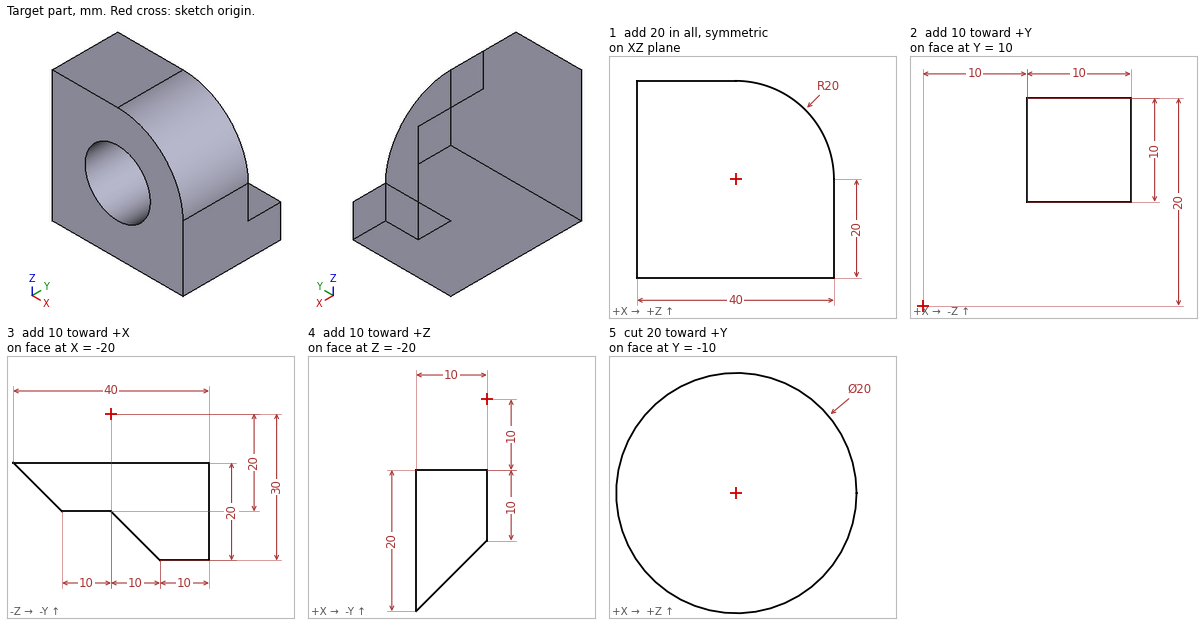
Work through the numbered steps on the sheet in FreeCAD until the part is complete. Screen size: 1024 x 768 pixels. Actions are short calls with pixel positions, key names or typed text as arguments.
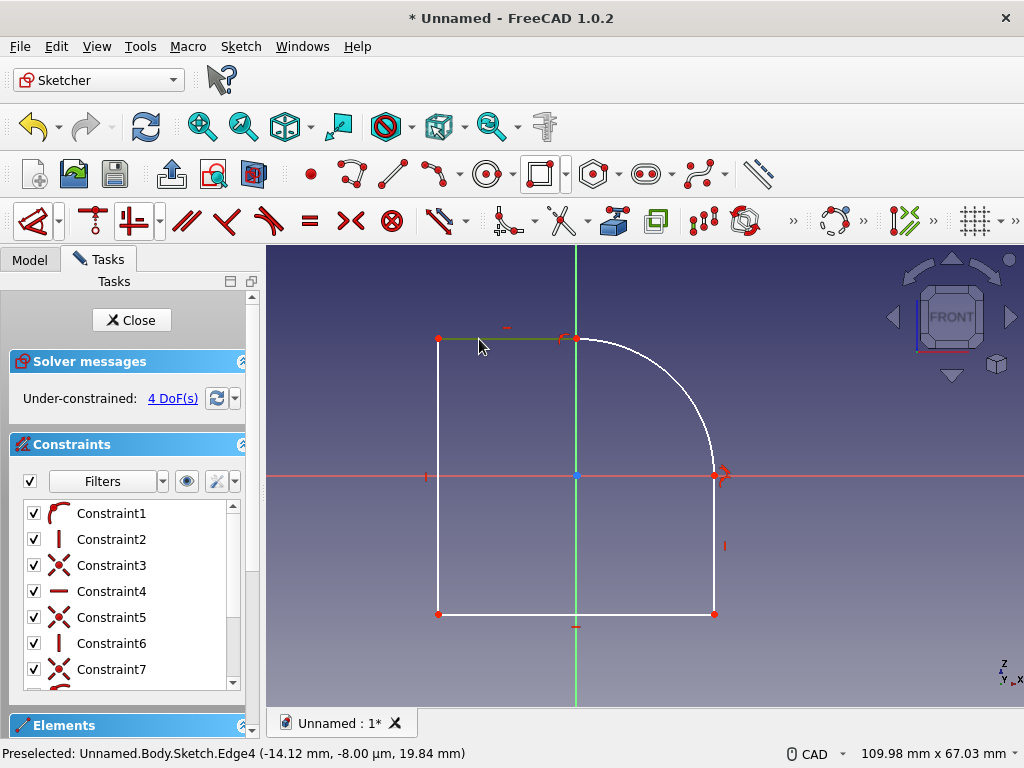
click(699, 413)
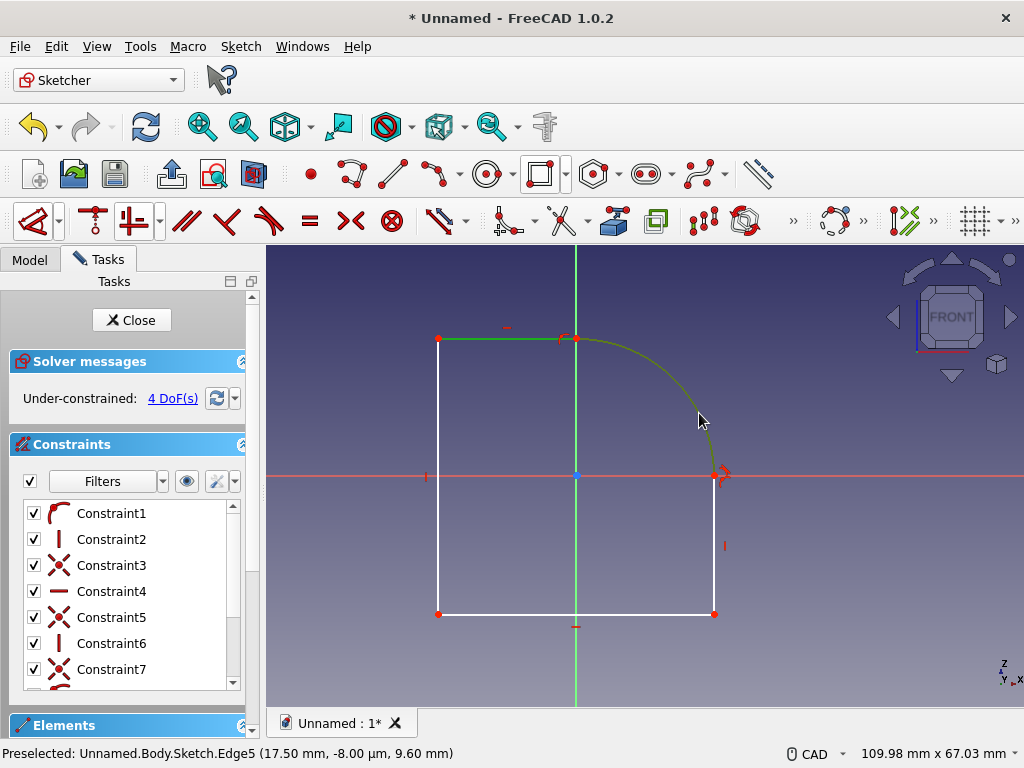
click(269, 222)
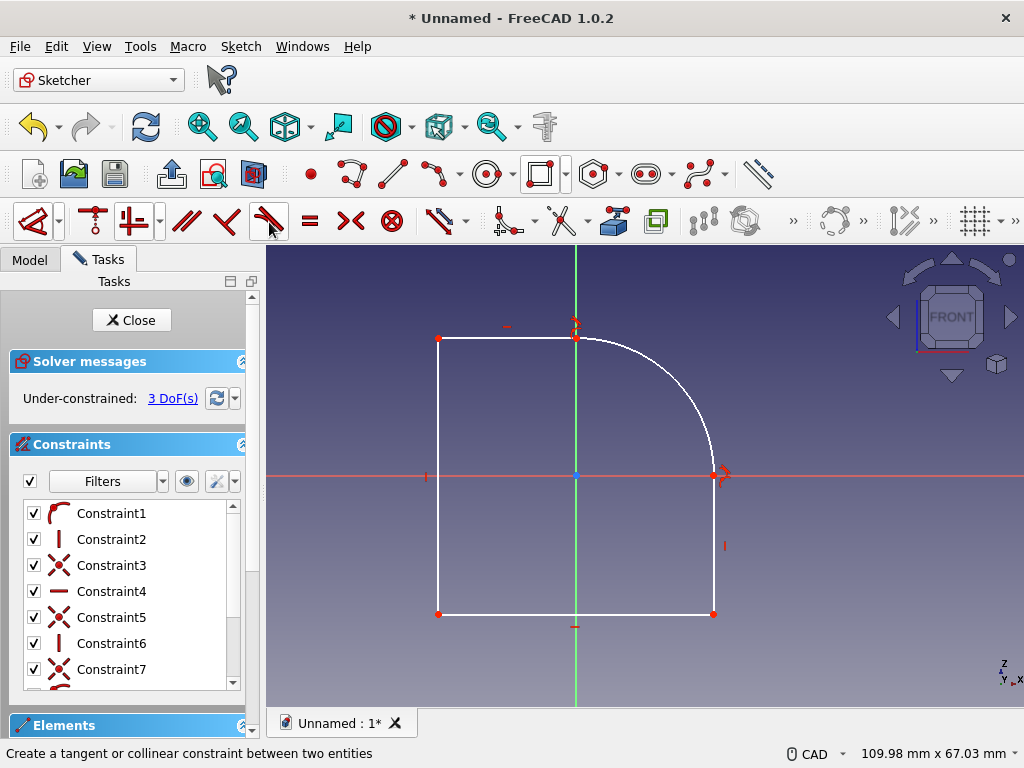
click(699, 413)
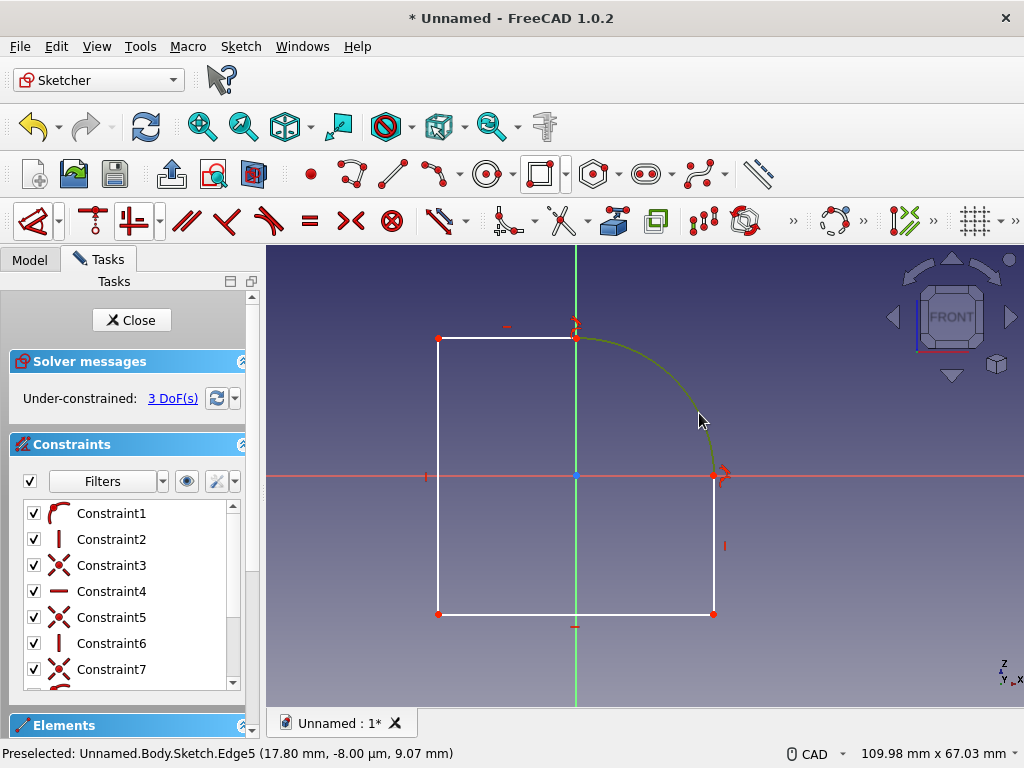
key(k)
key(r)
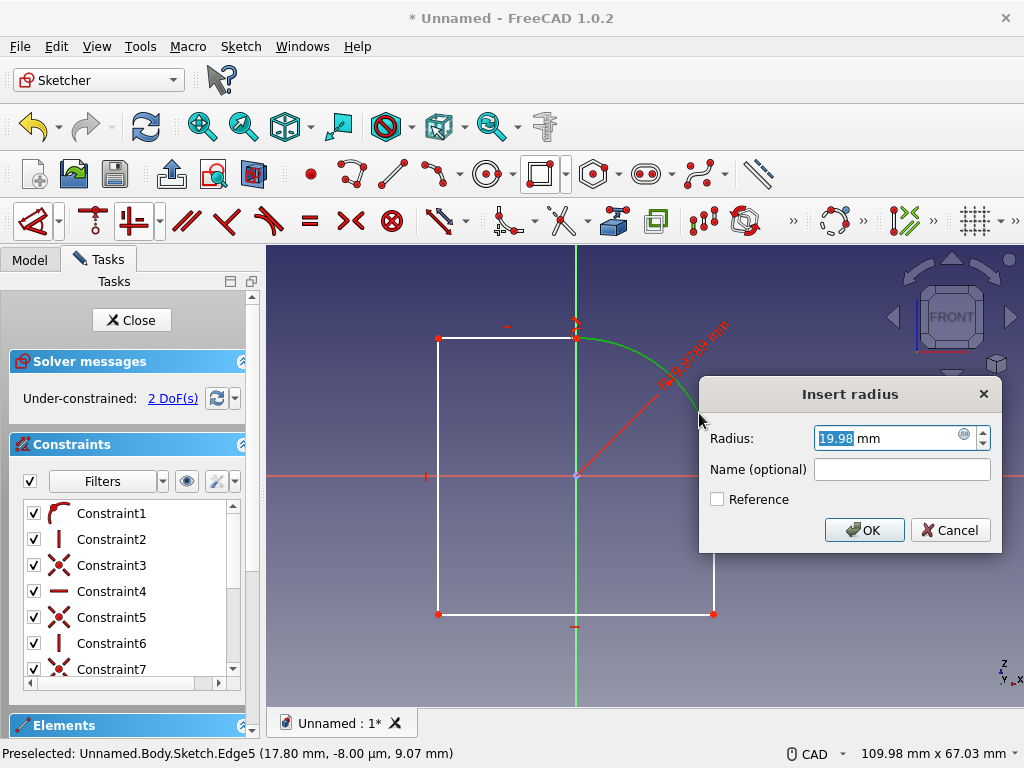
text(20)
key(Return)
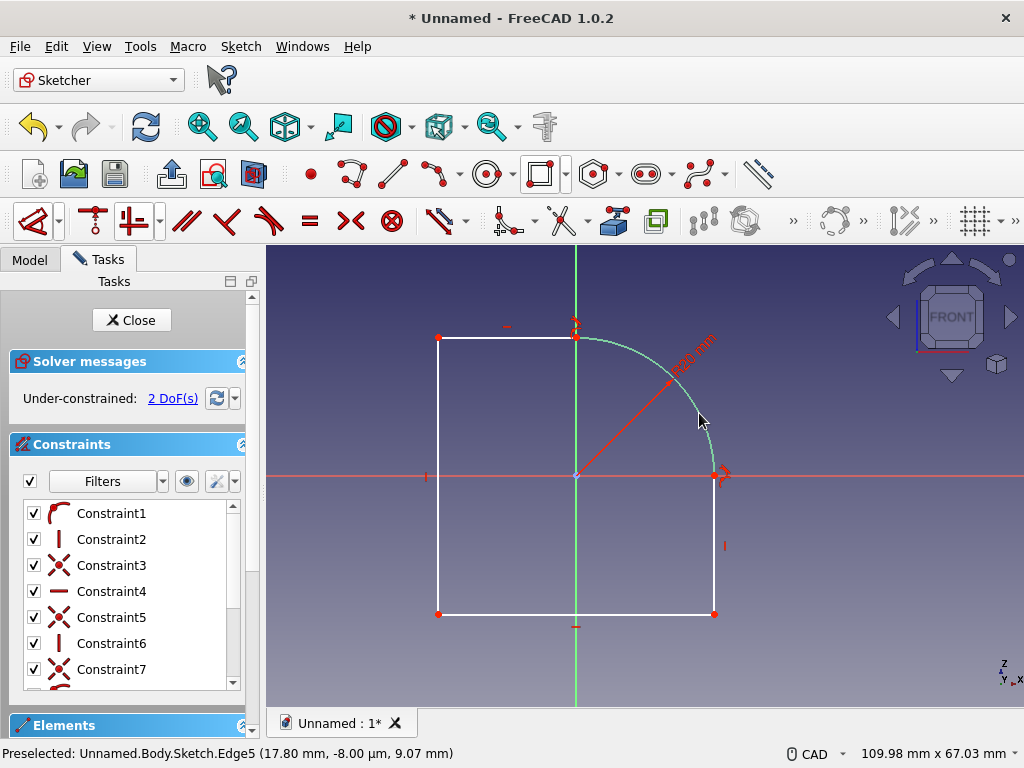
click(714, 518)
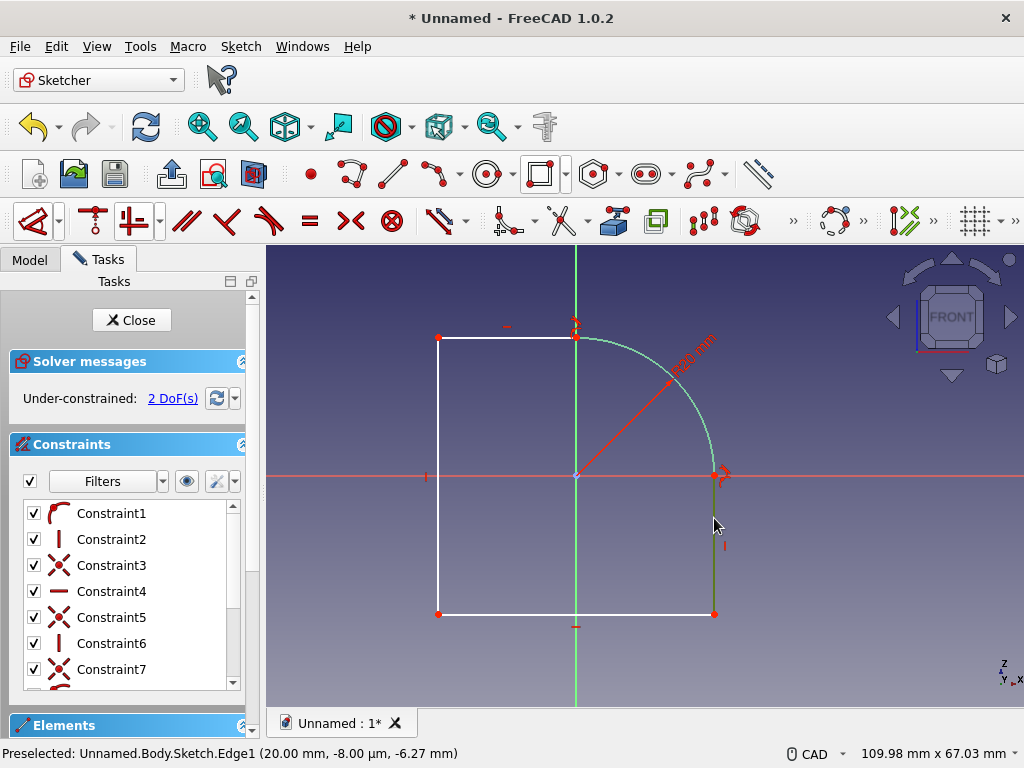
click(58, 222)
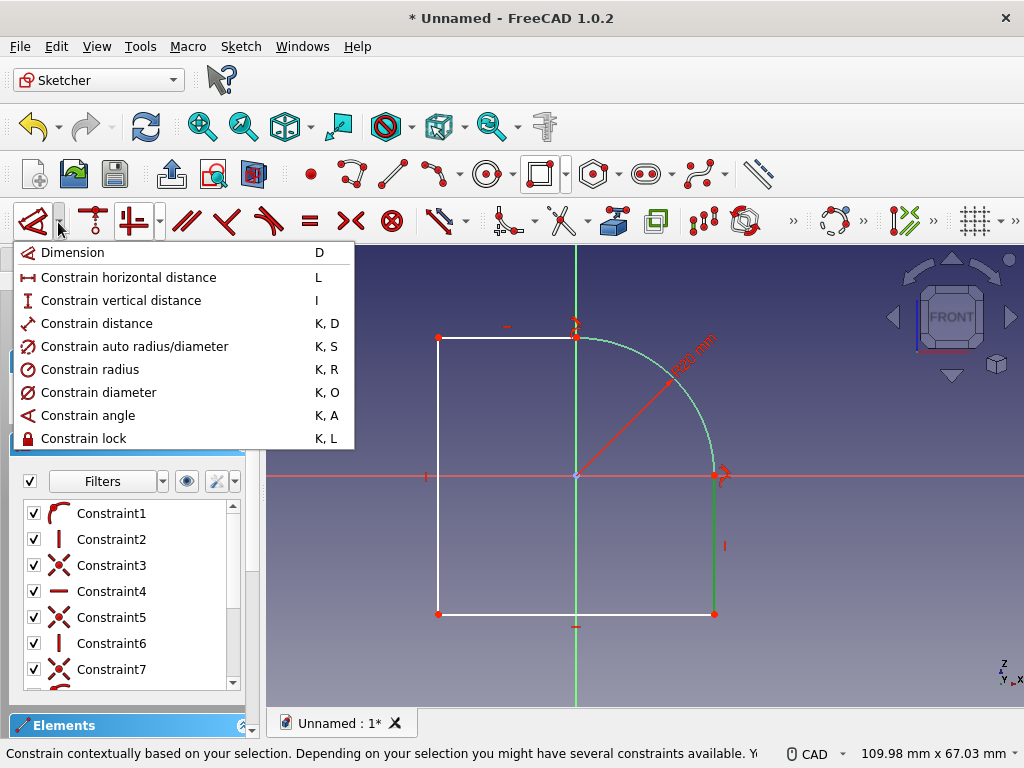
click(184, 300)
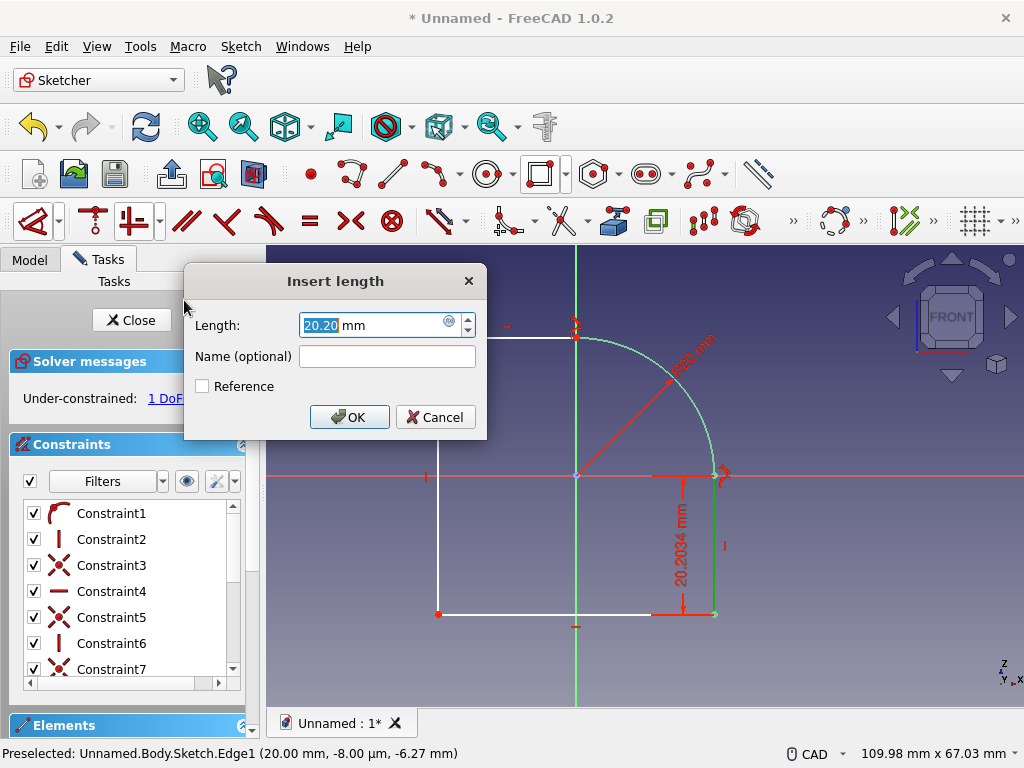
text(20)
key(Return)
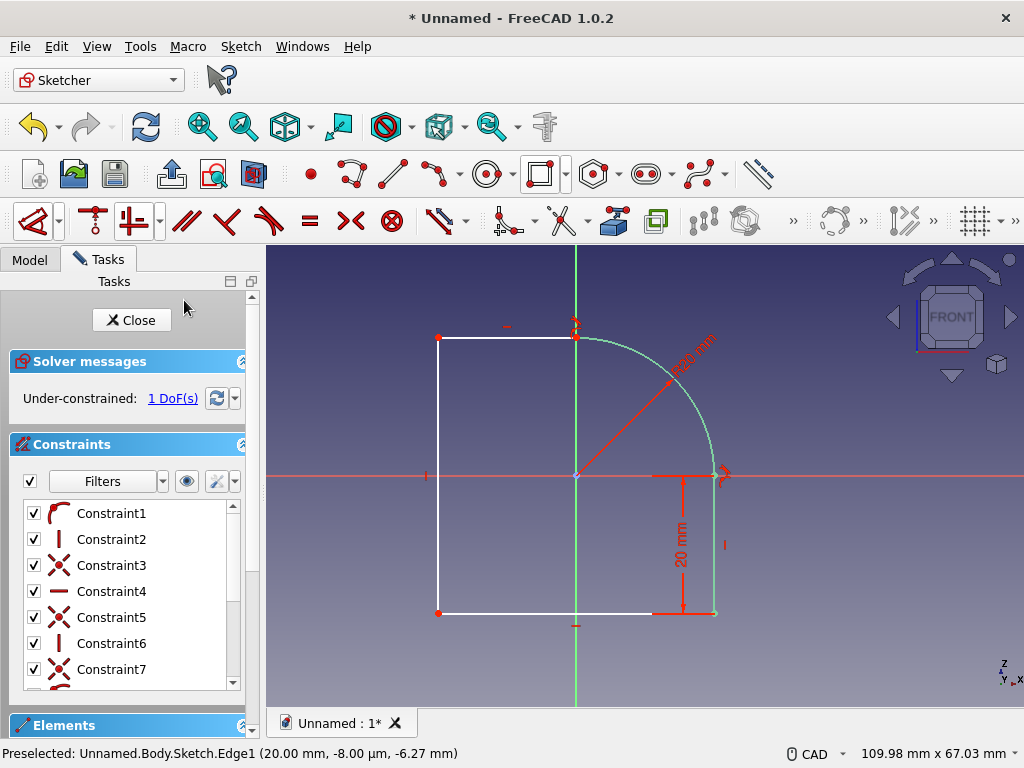
click(631, 614)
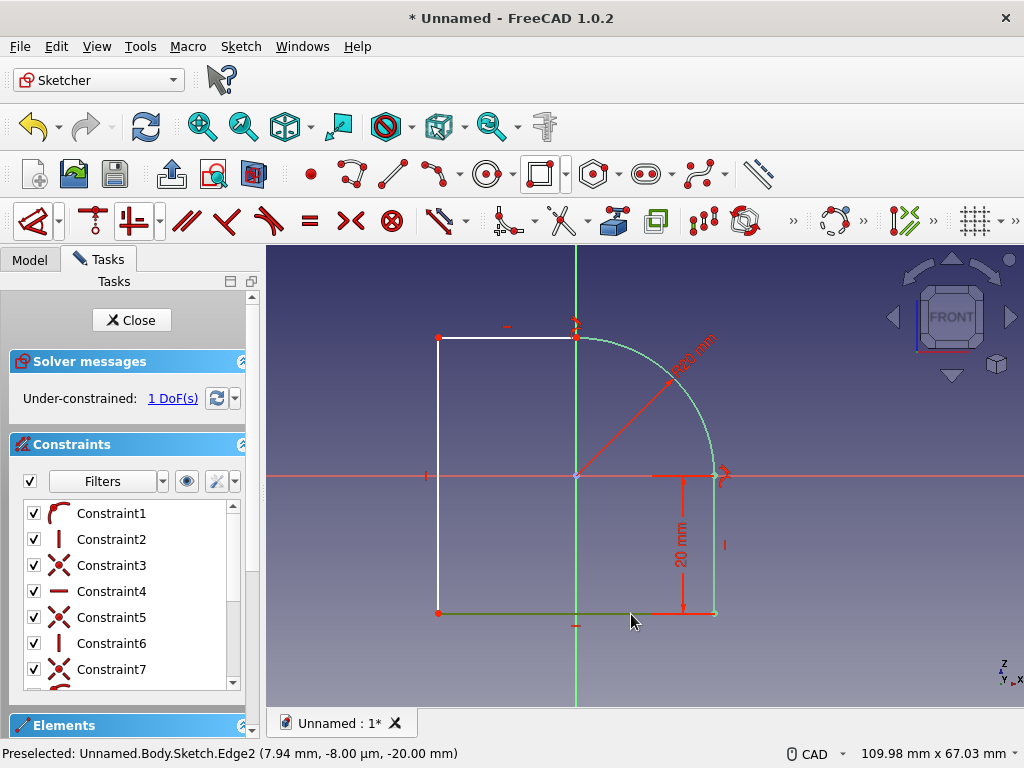
click(58, 222)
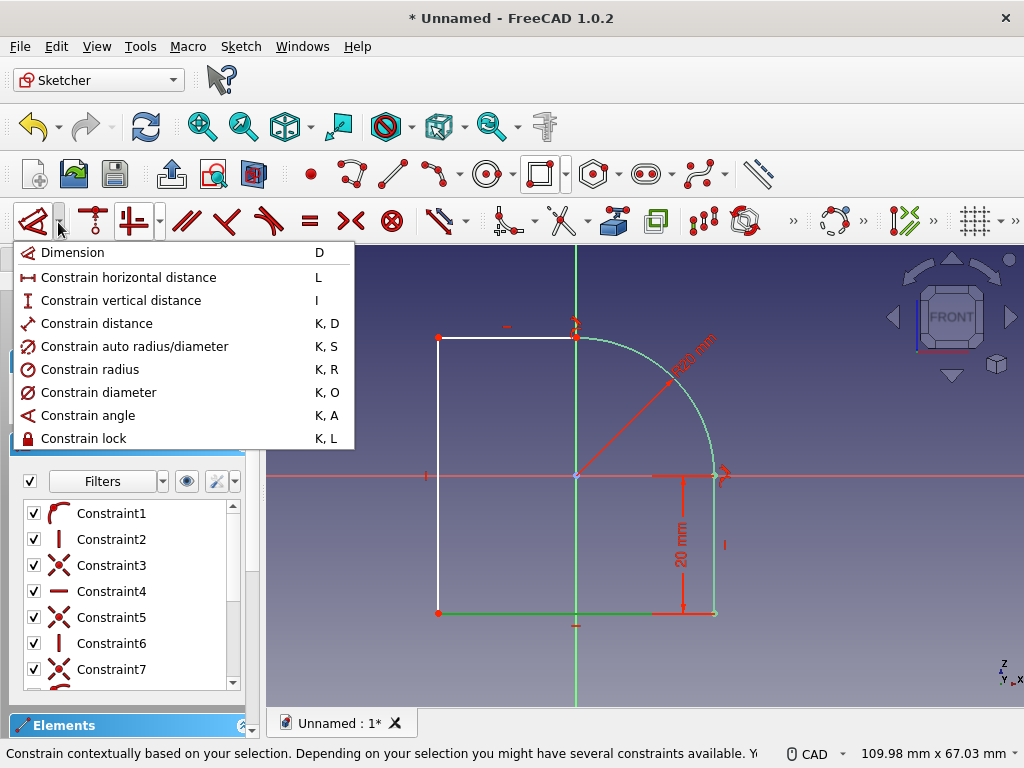
click(184, 278)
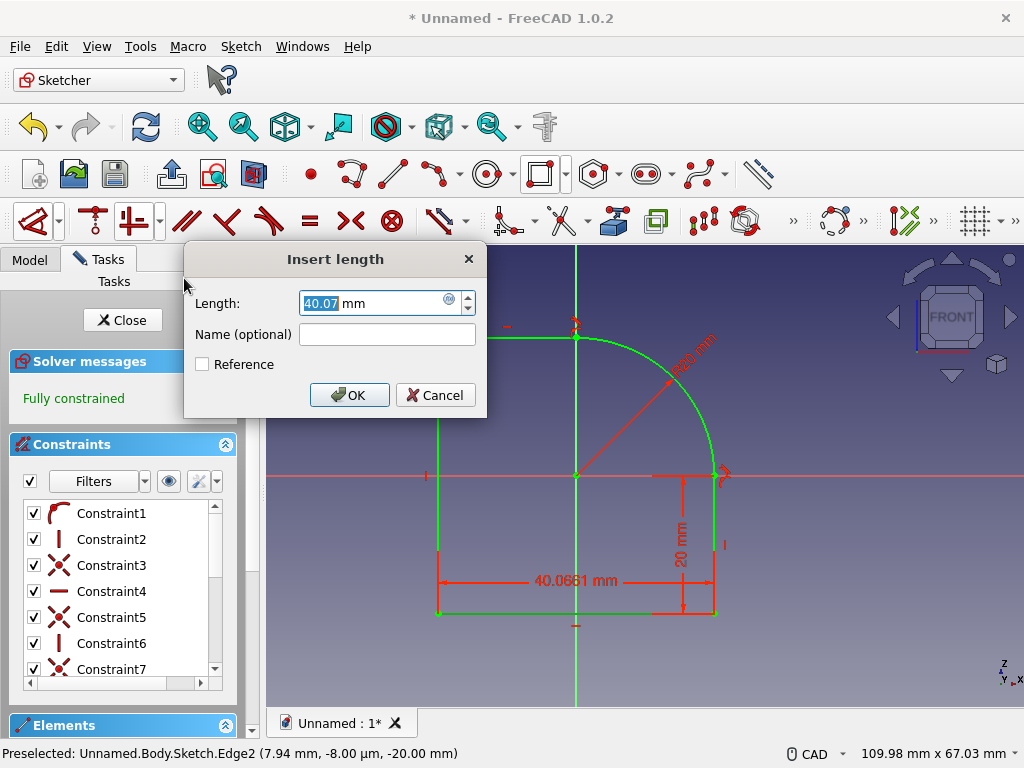
text(40)
key(Return)